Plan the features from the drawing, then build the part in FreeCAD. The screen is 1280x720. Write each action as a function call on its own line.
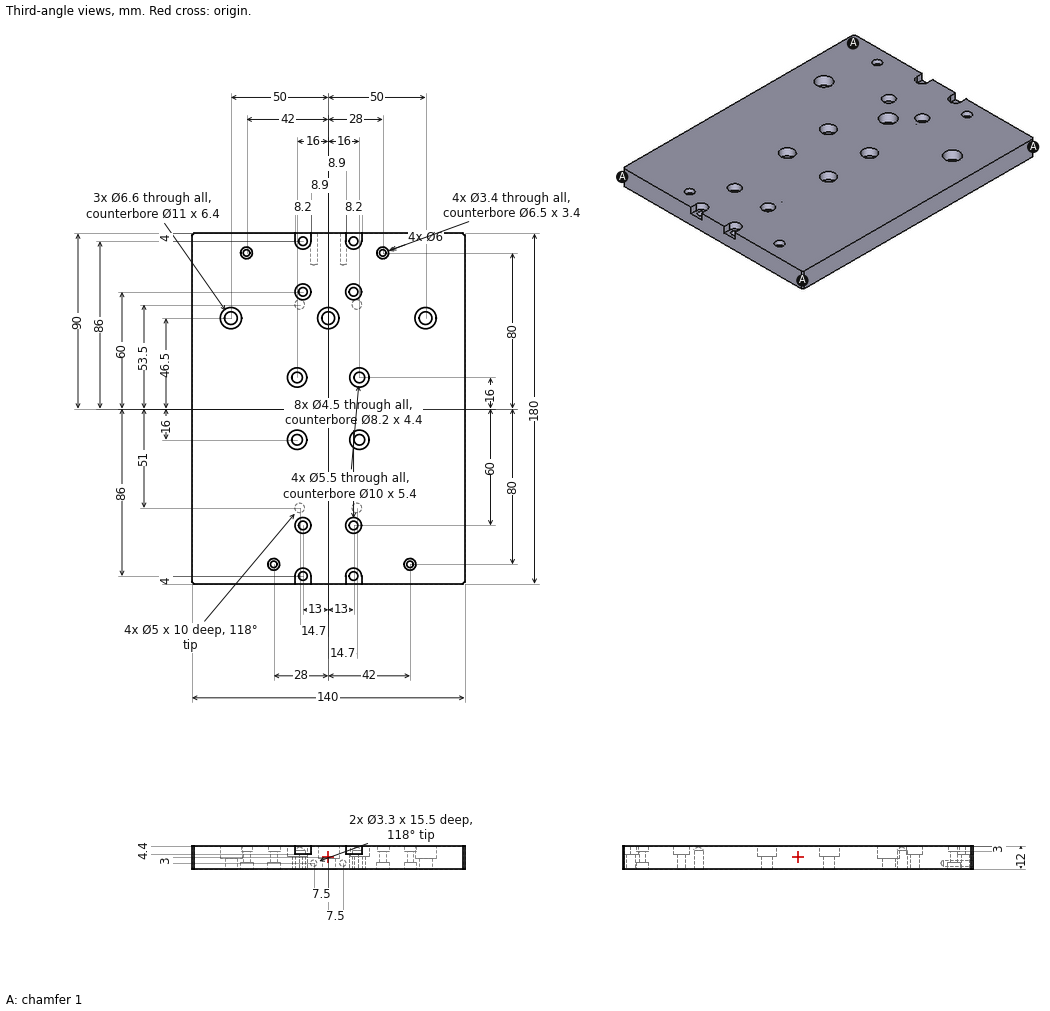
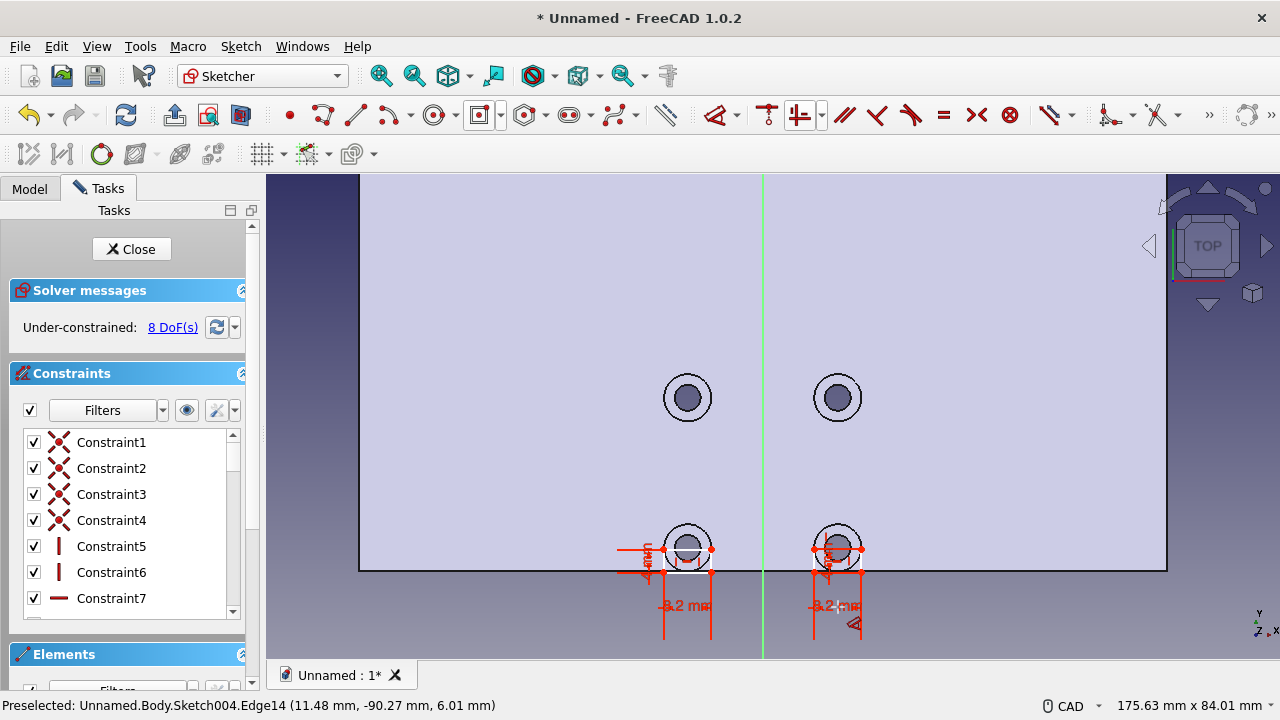
scroll(679, 574, down, 6)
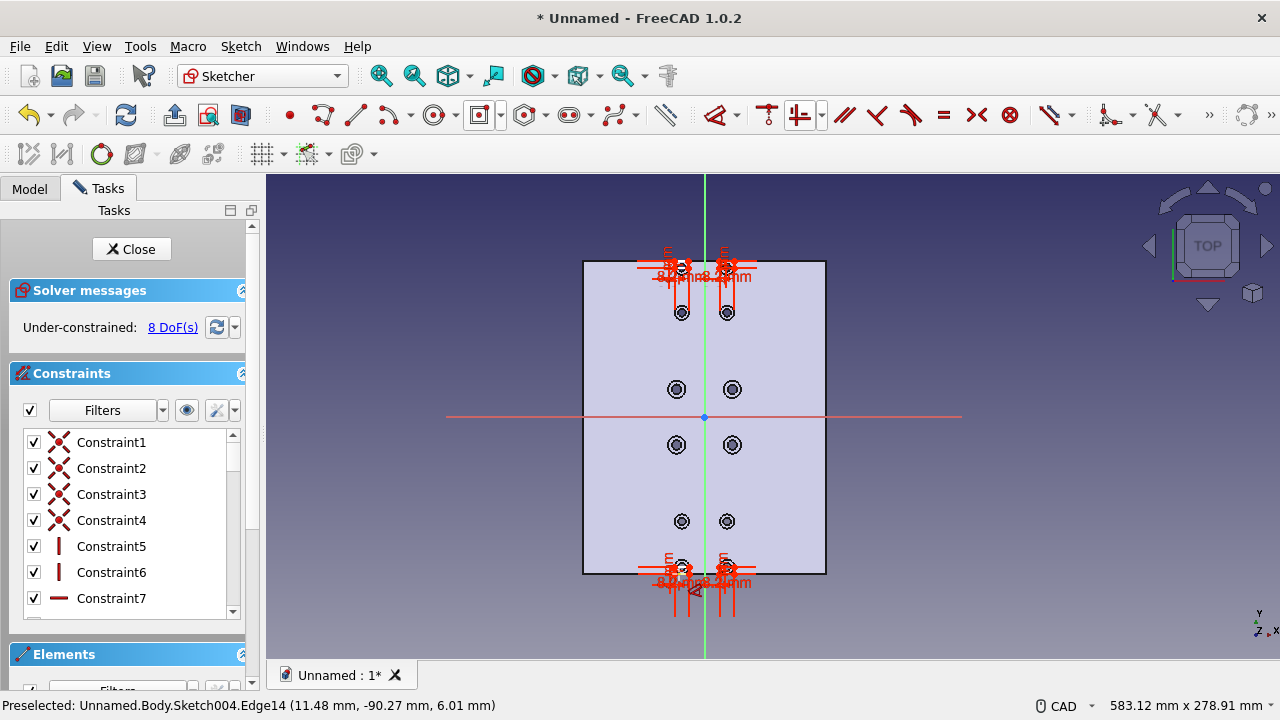
scroll(675, 261, up, 3)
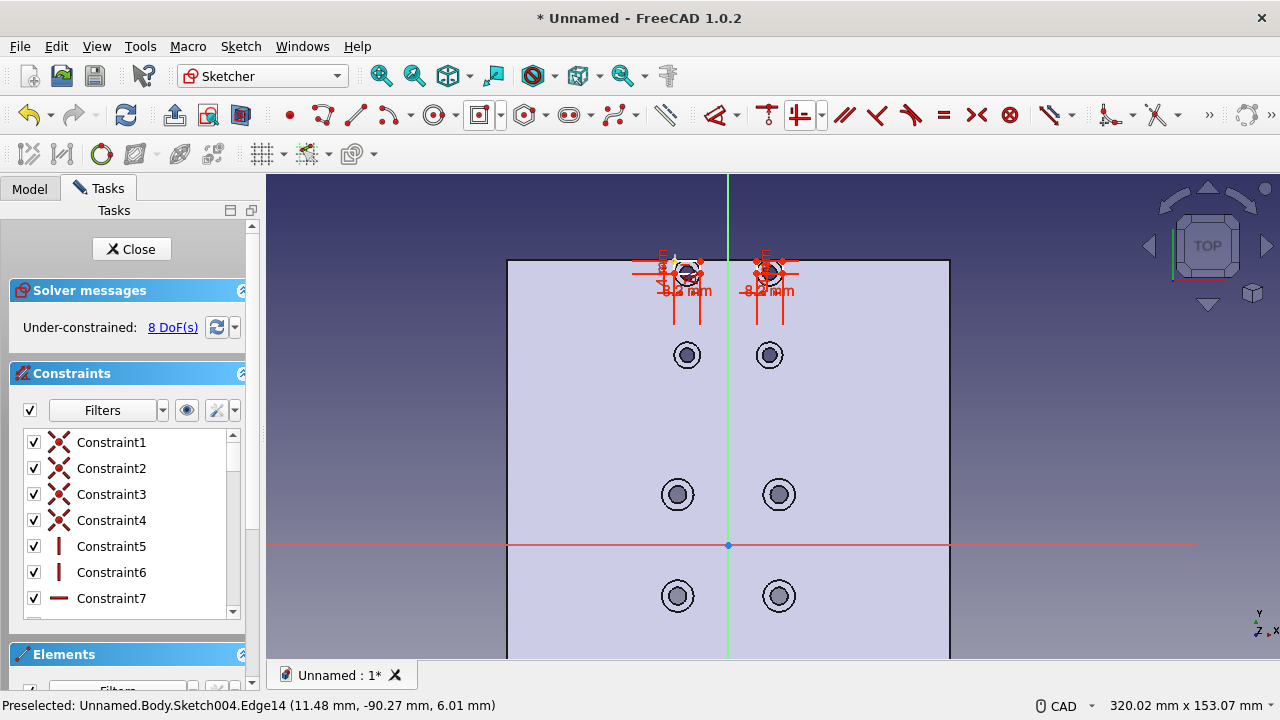
click(674, 261)
click(640, 403)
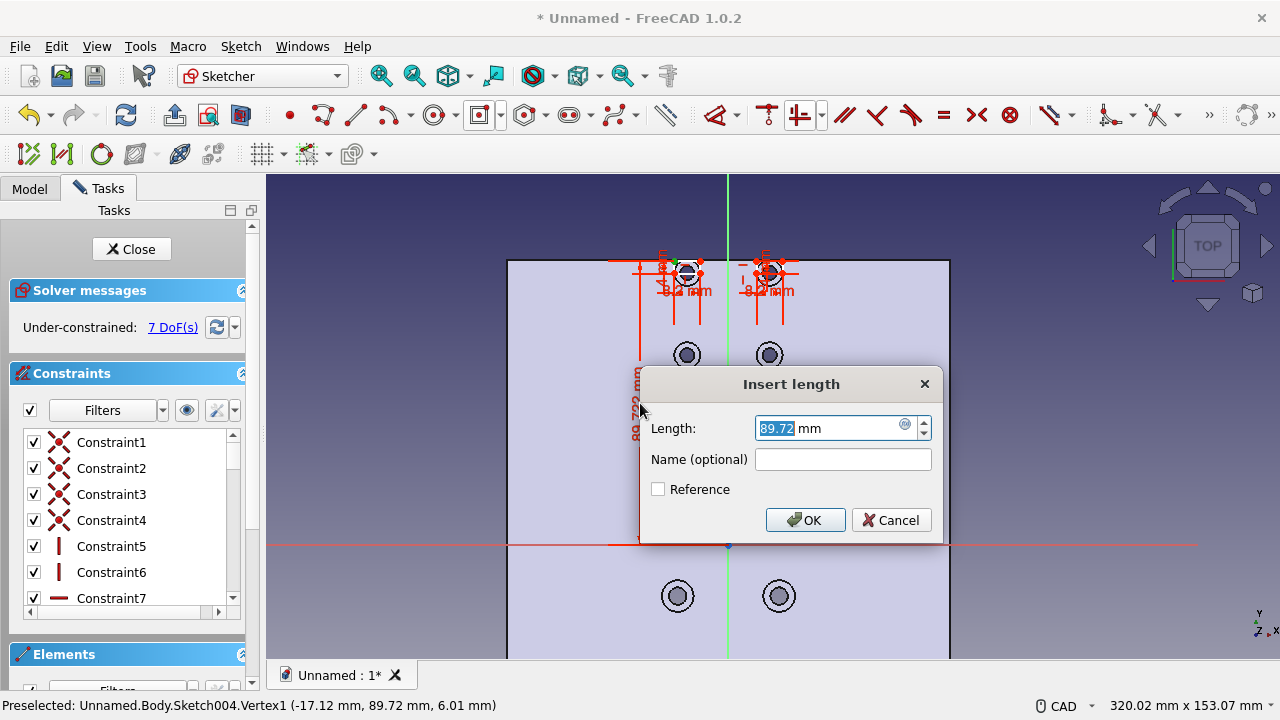
text(90)
key(Return)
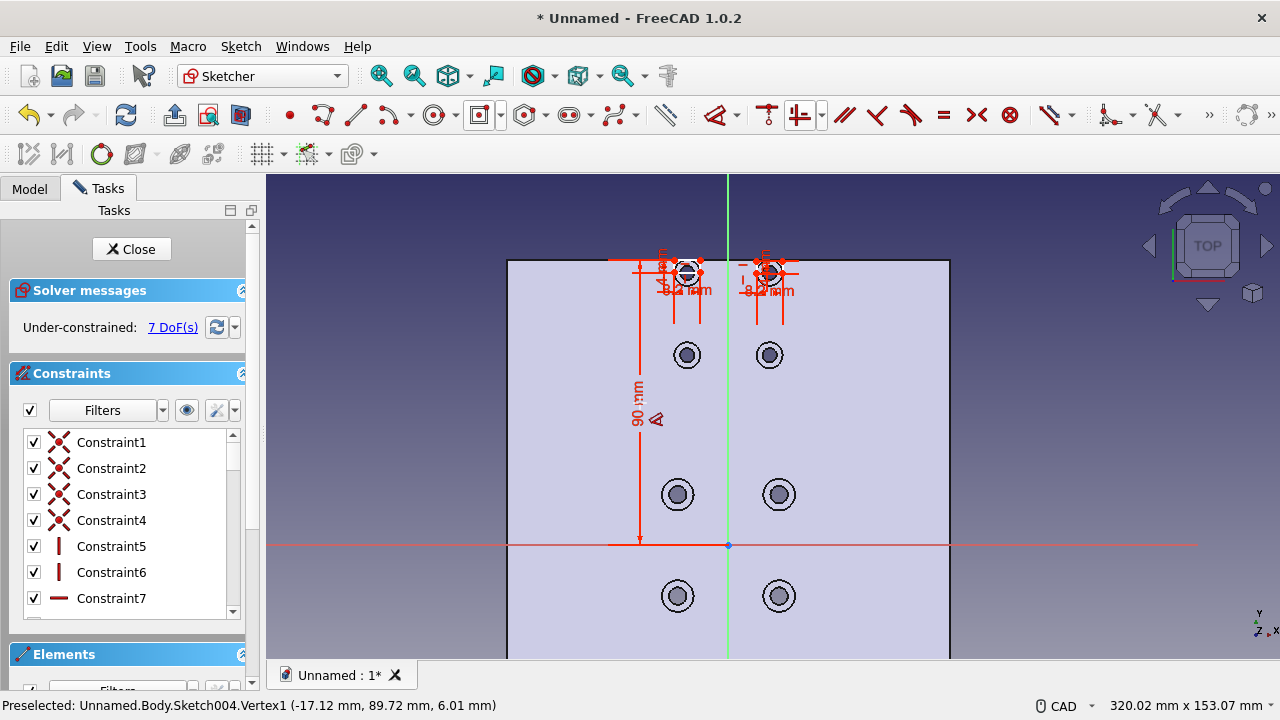
click(757, 261)
click(791, 403)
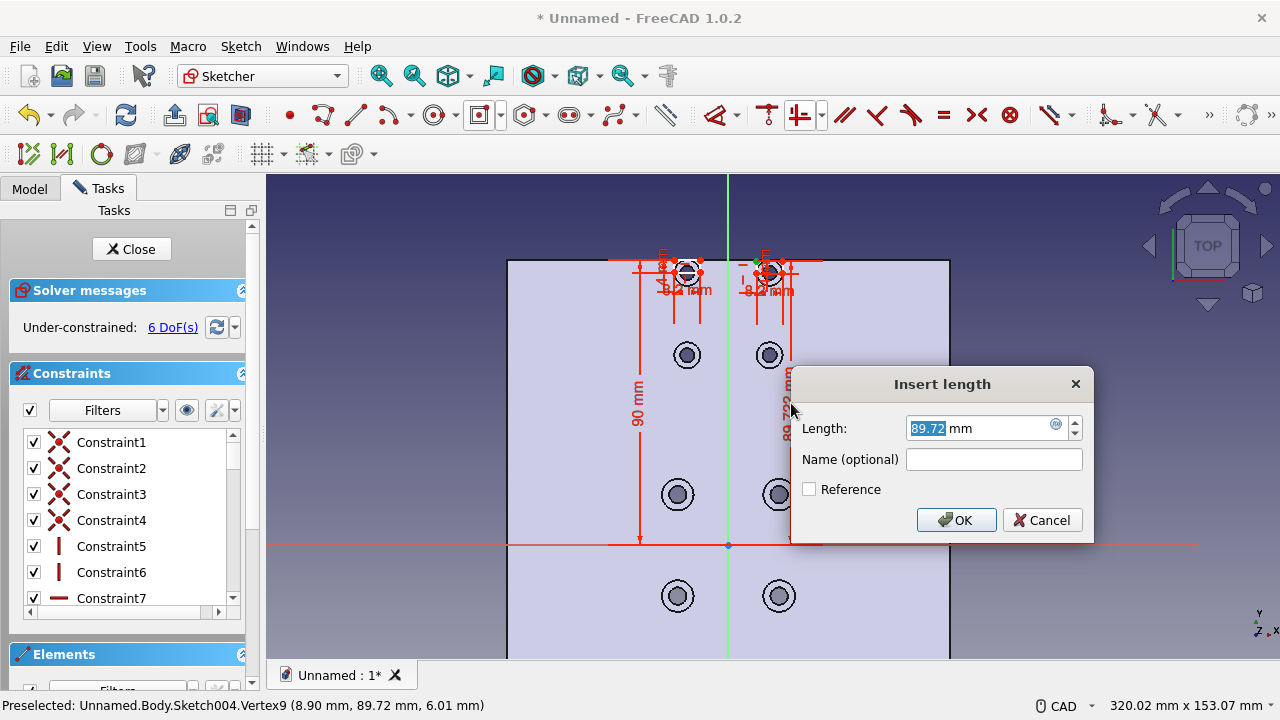
text(90)
key(Return)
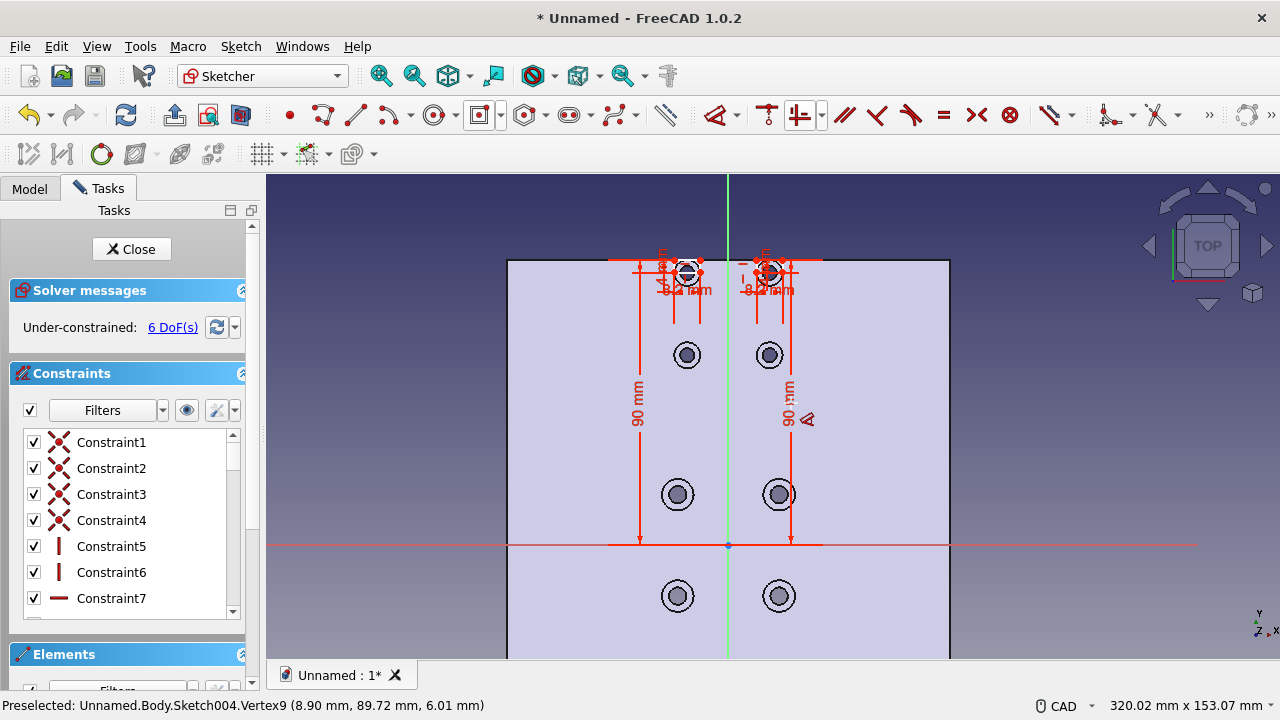
scroll(675, 260, down, 3)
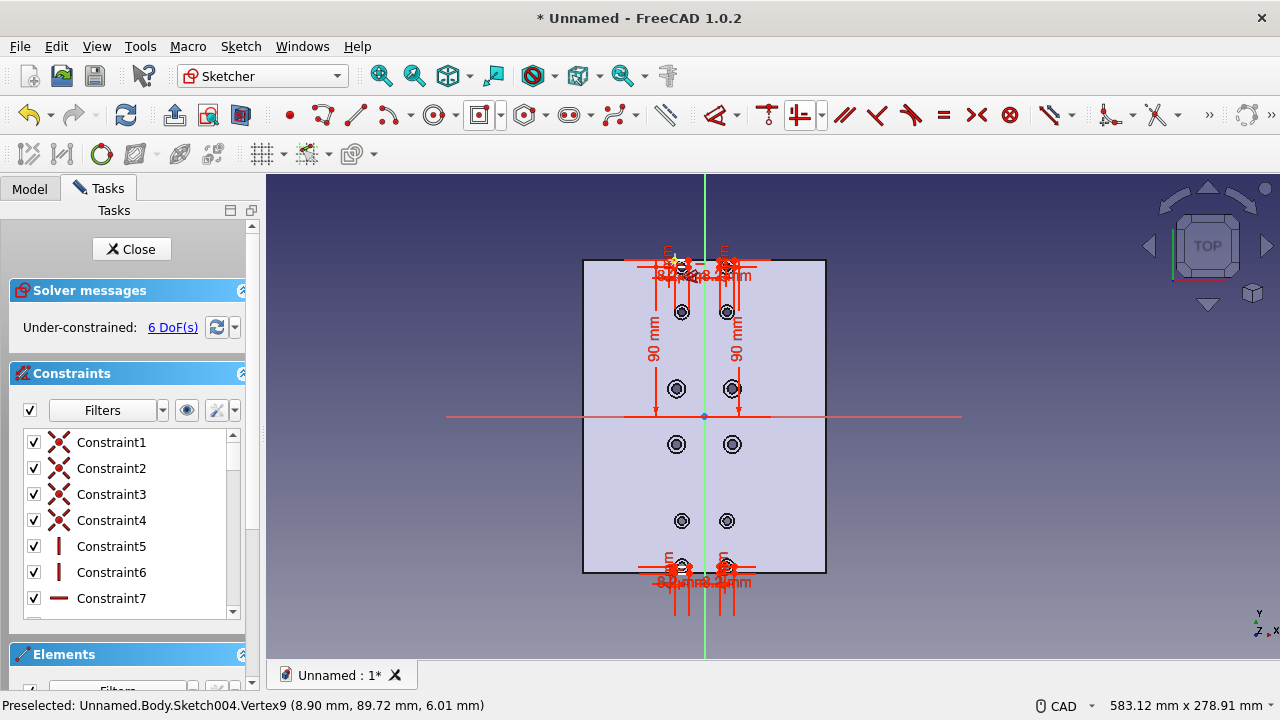
scroll(675, 567, up, 3)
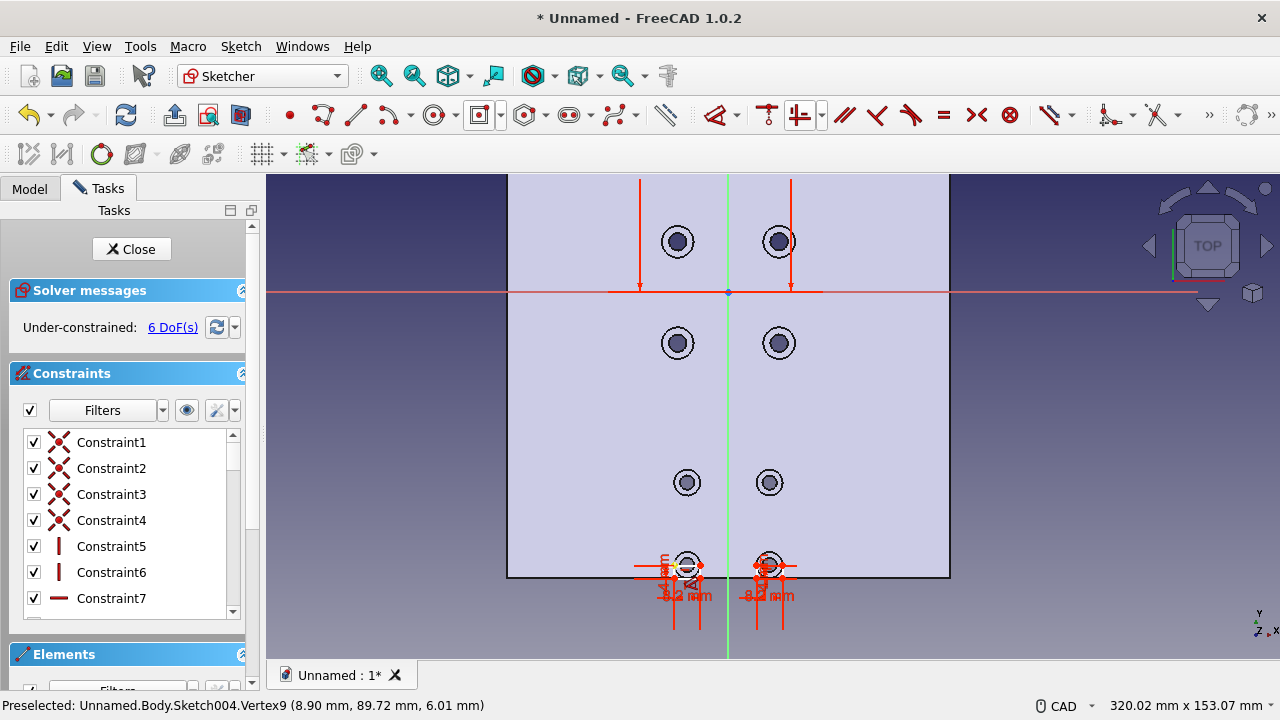
click(674, 566)
click(640, 429)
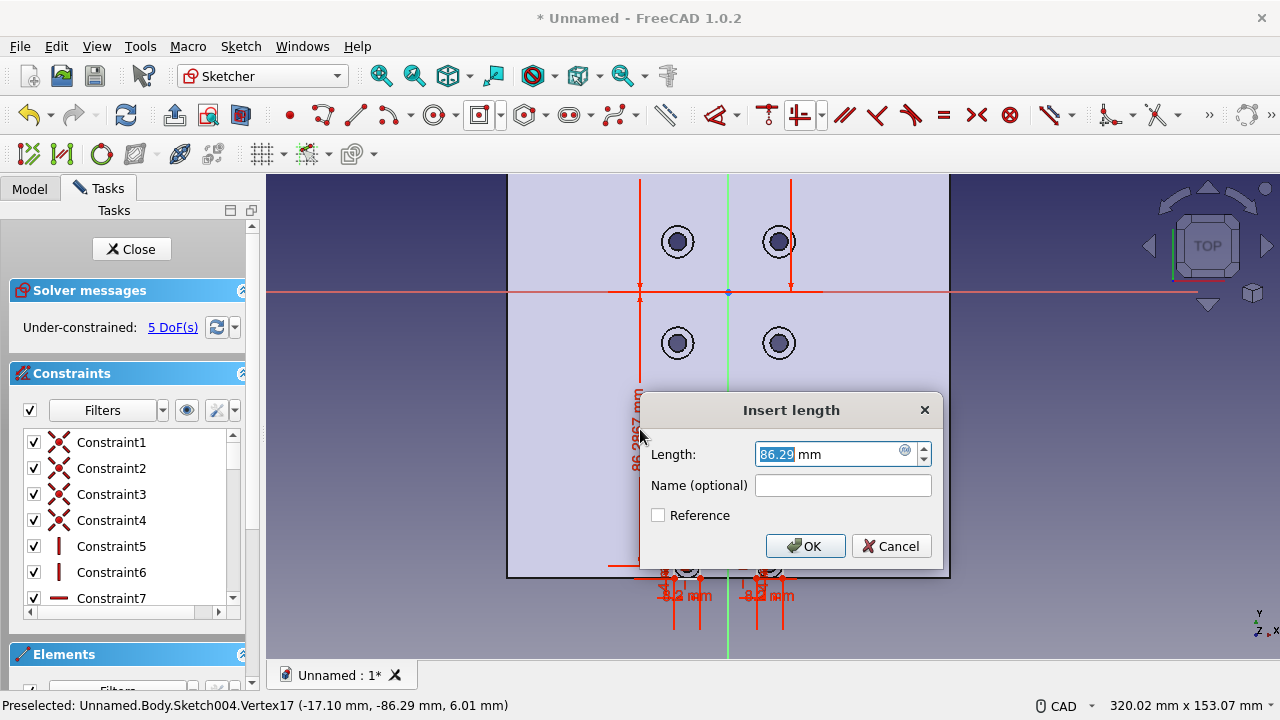
text(86)
key(Return)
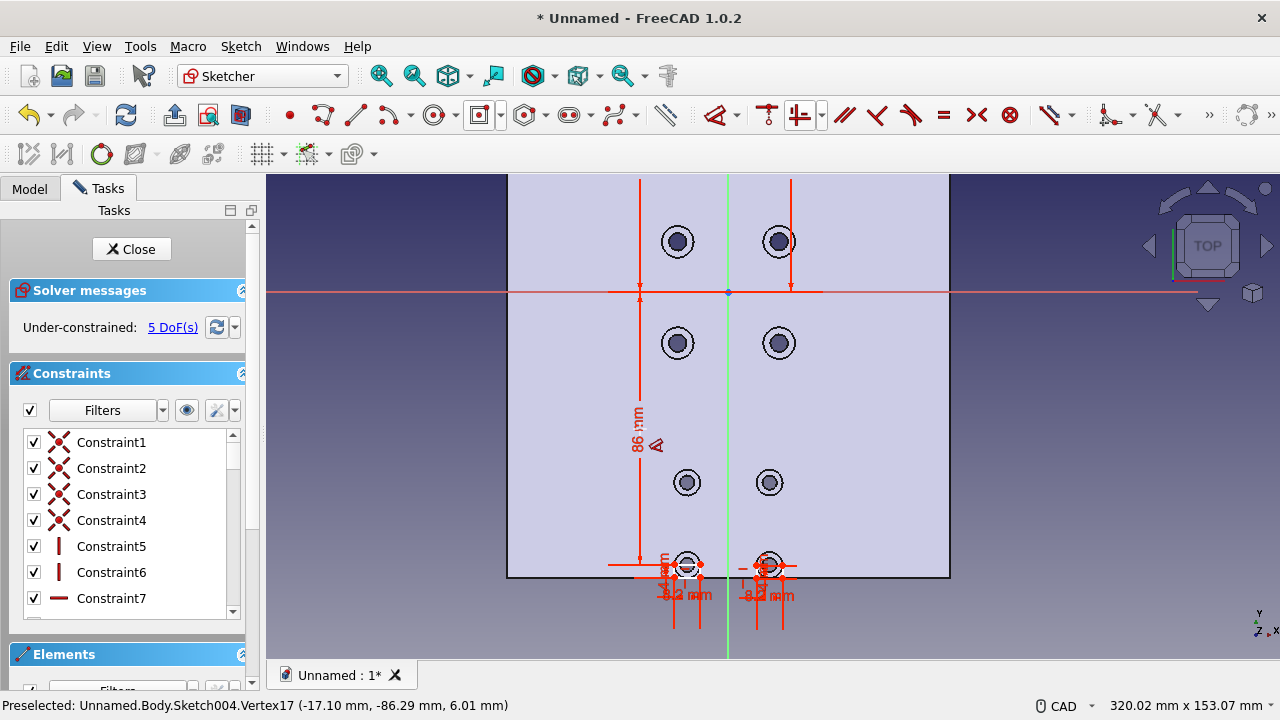
click(757, 566)
click(791, 429)